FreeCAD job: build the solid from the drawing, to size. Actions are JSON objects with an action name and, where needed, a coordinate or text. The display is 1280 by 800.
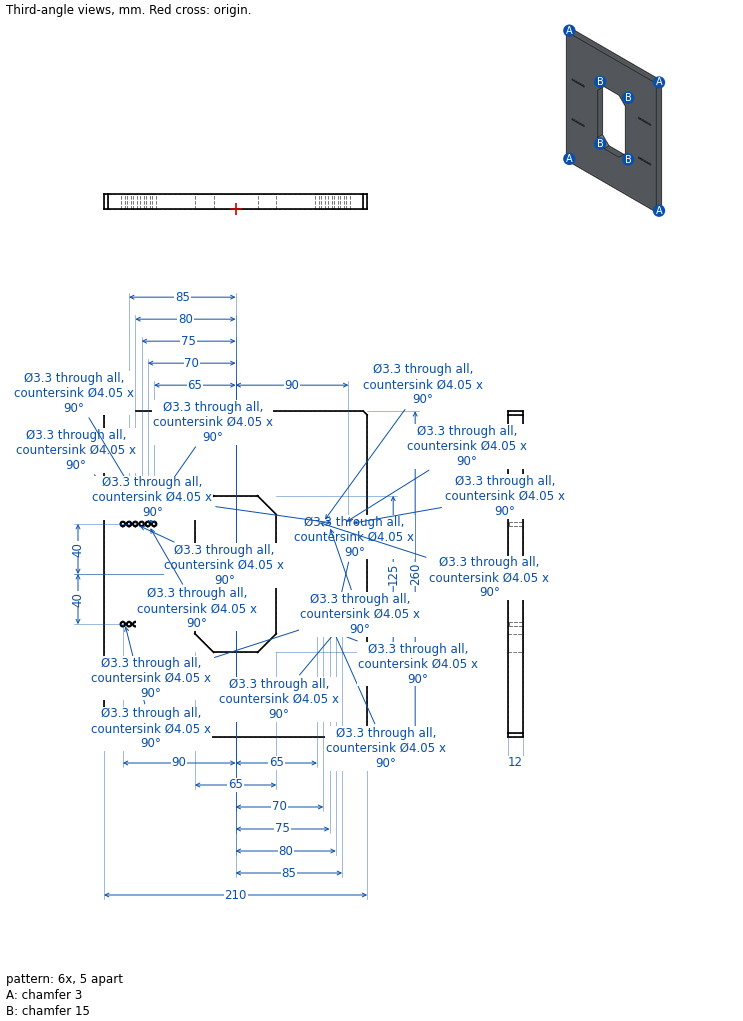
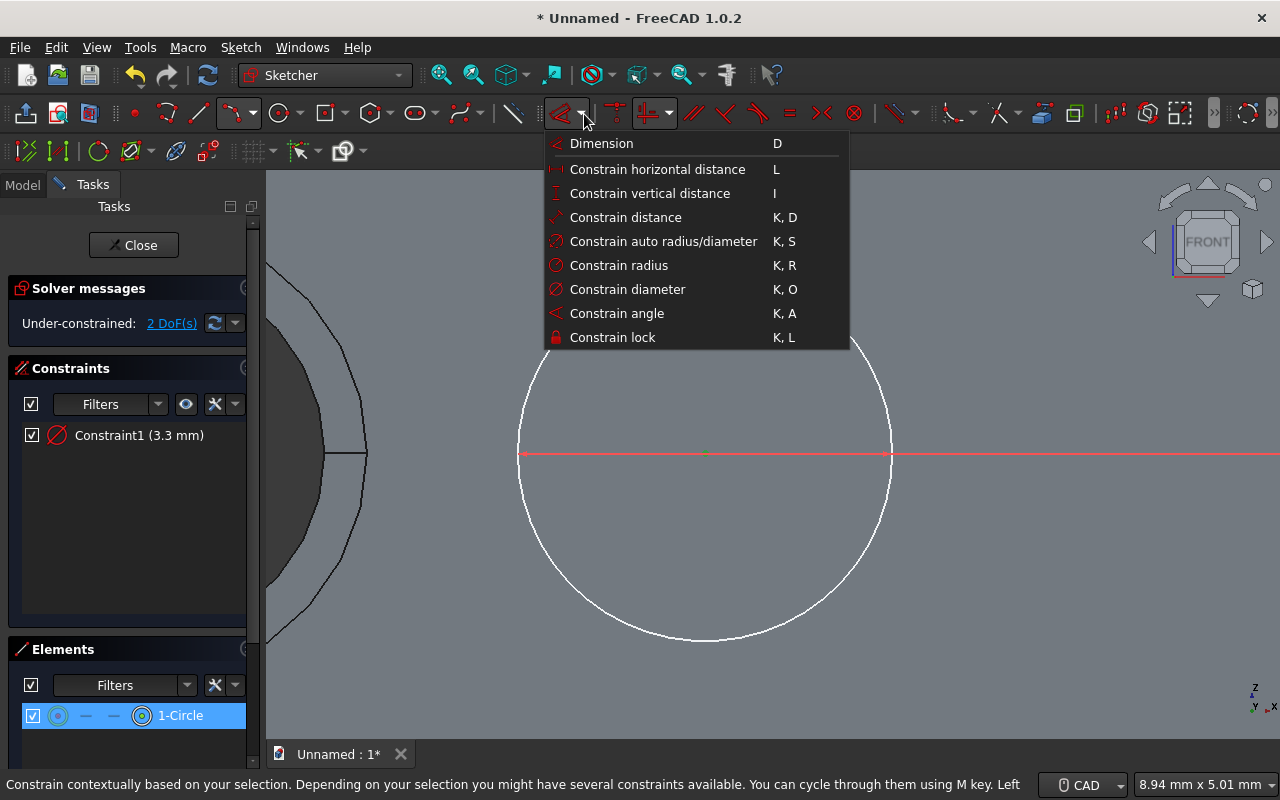
{"action": "left_click", "coordinate": [697, 169]}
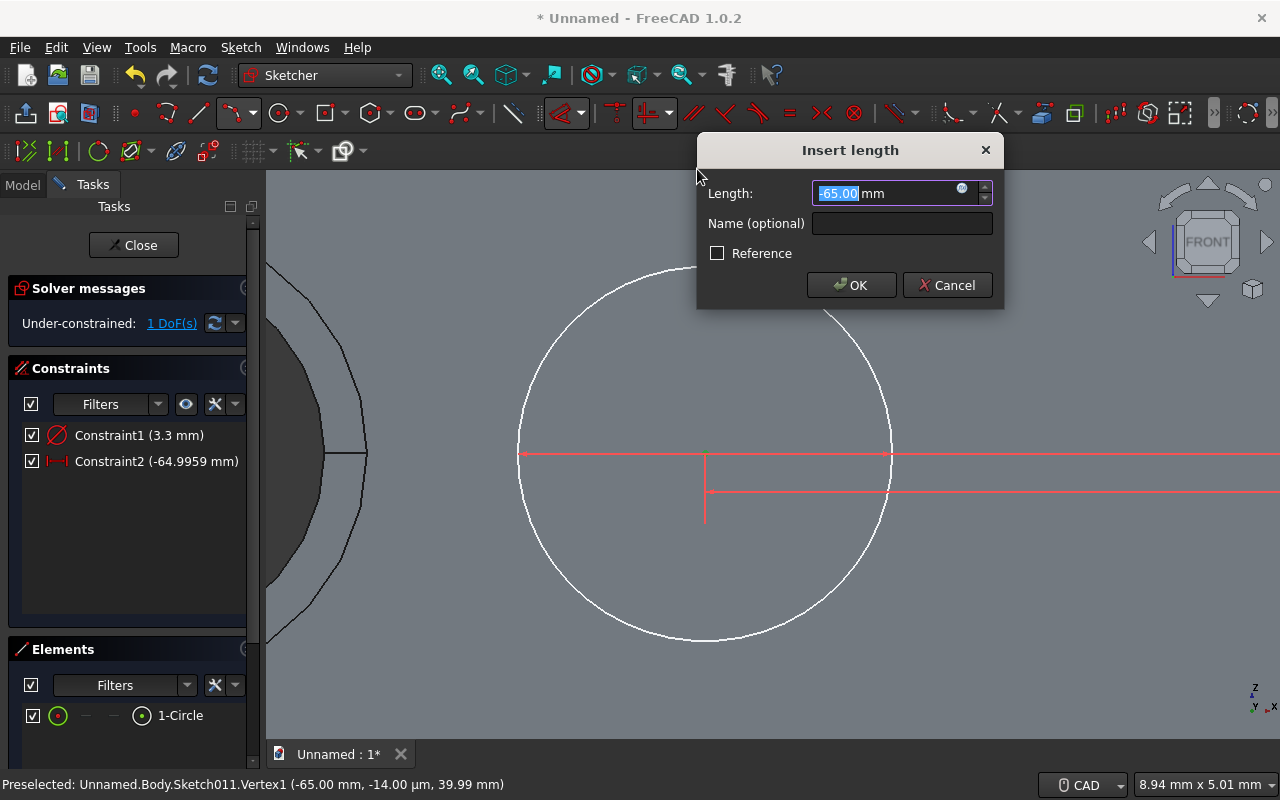
{"action": "type", "text": "-65"}
{"action": "key", "text": "Return"}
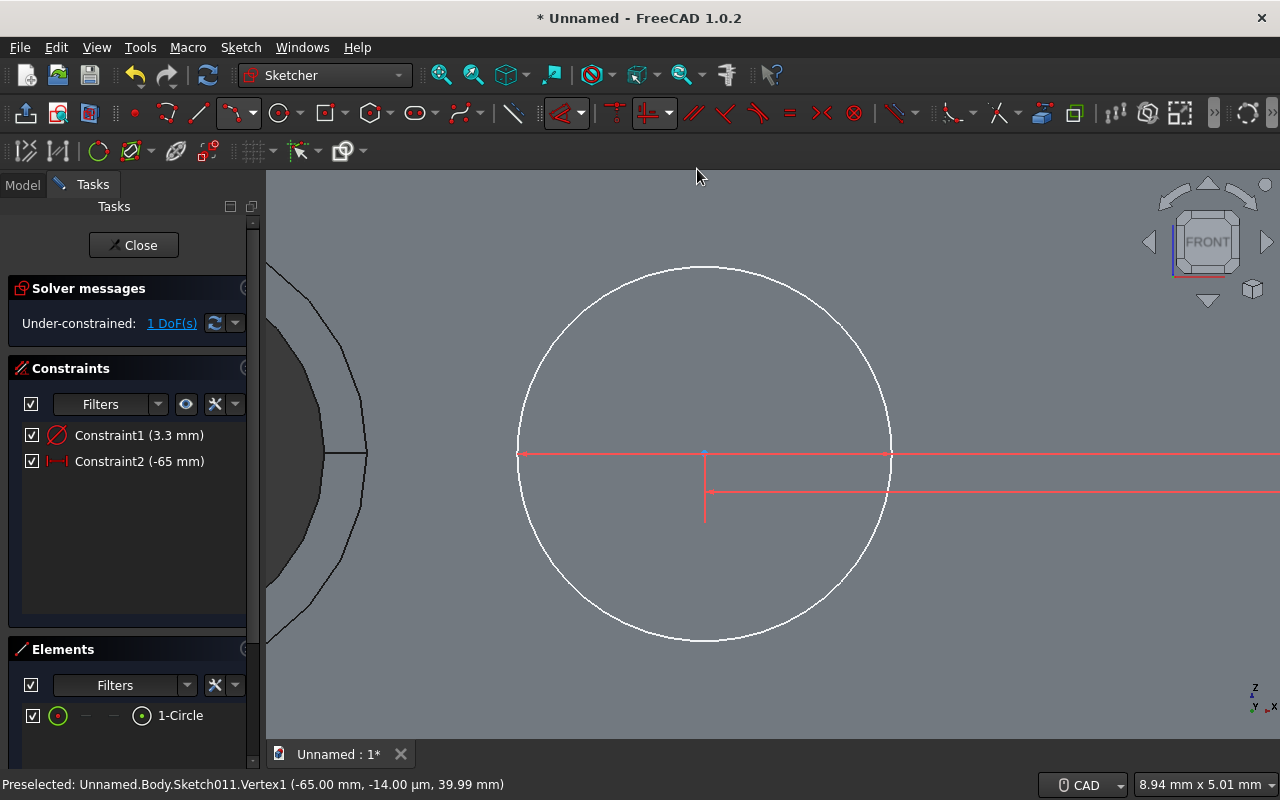
{"action": "left_click", "coordinate": [705, 454]}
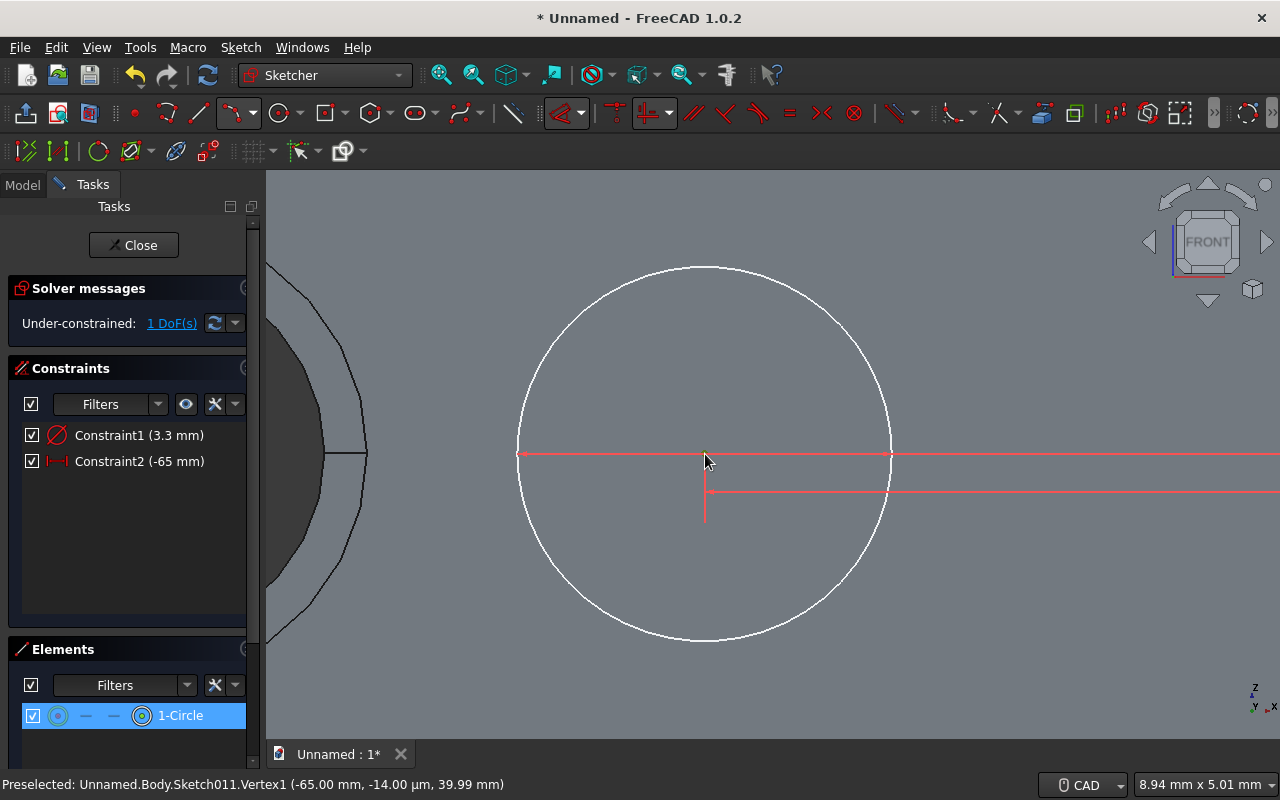
{"action": "left_click", "coordinate": [584, 114]}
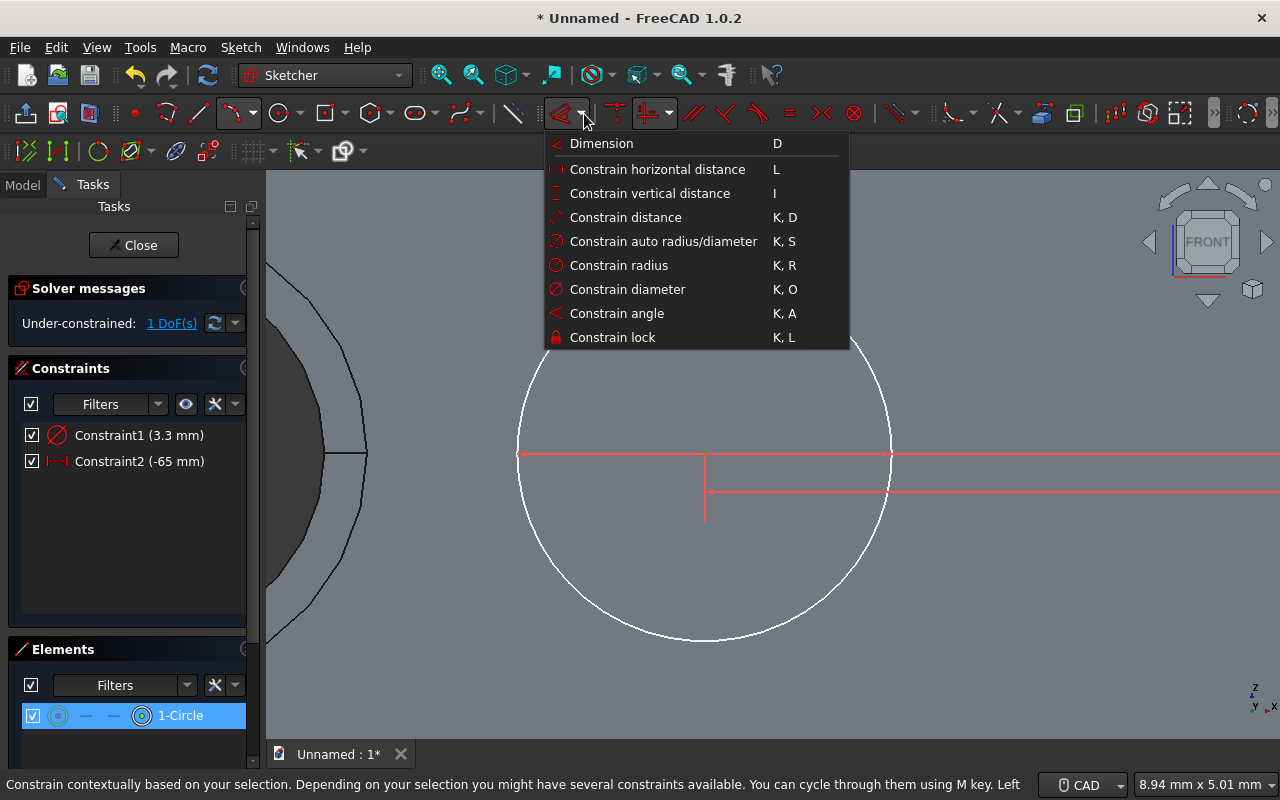
{"action": "left_click", "coordinate": [697, 193]}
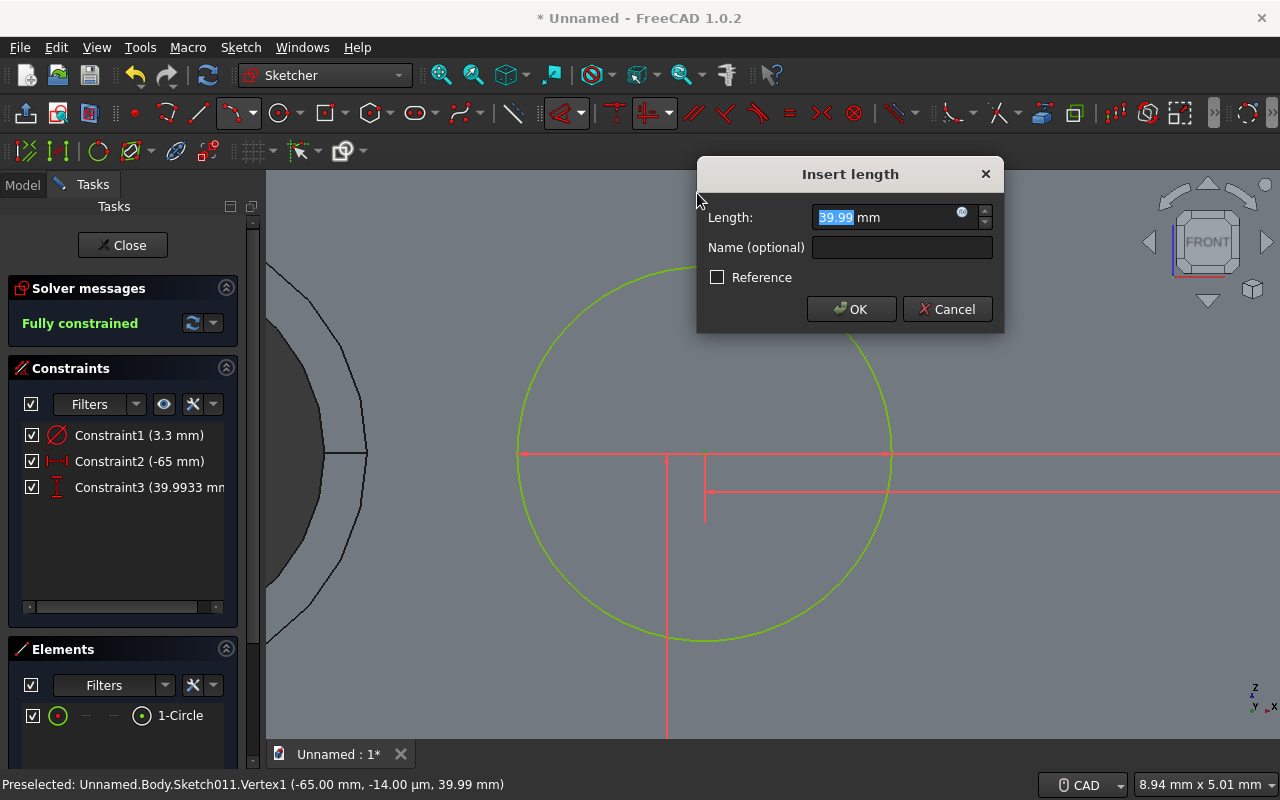
{"action": "type", "text": "40"}
{"action": "key", "text": "Return"}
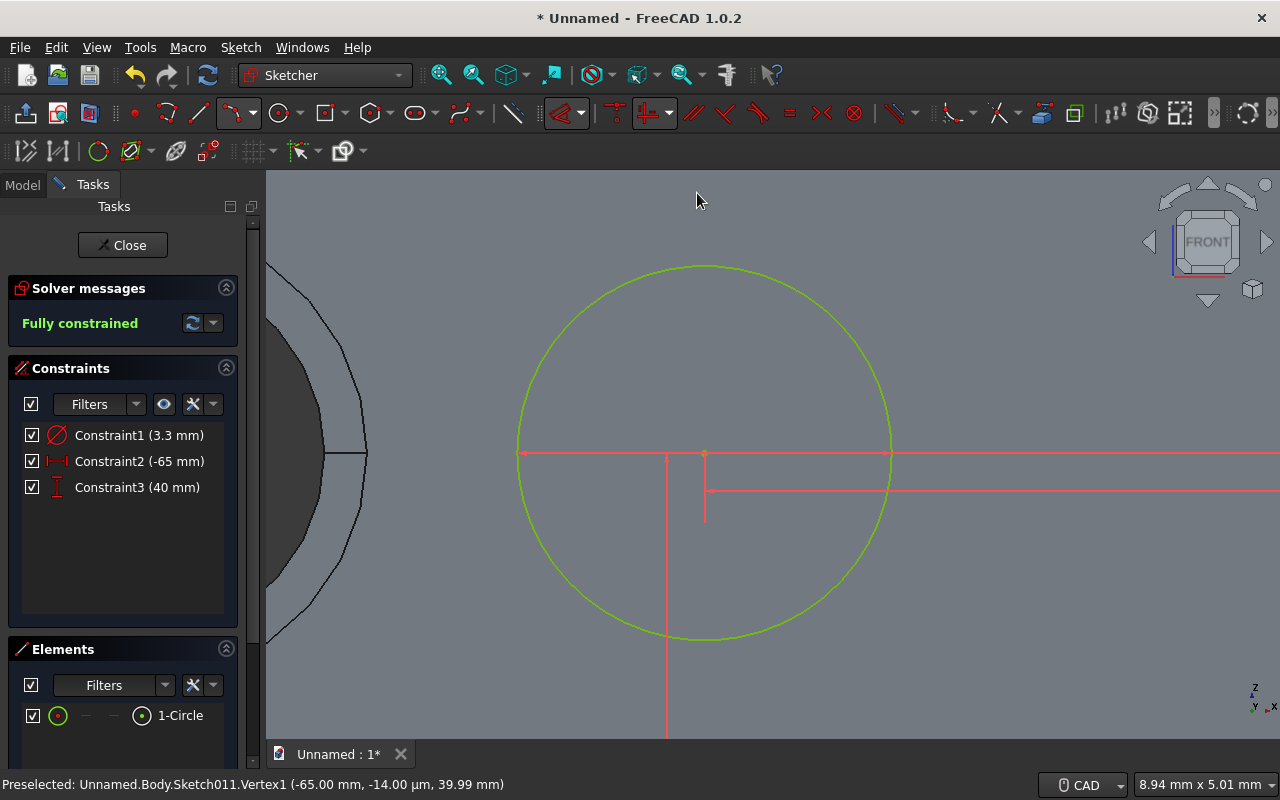
{"action": "left_click", "coordinate": [123, 245]}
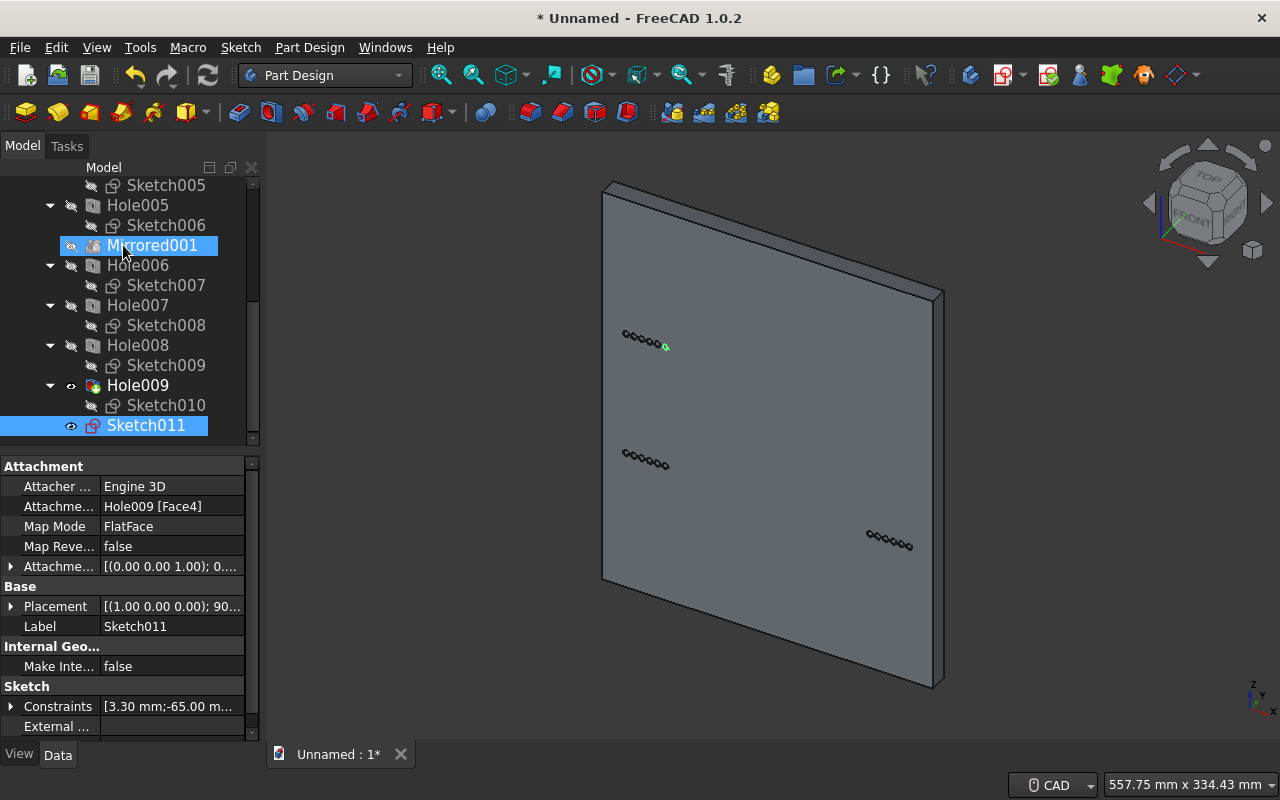
{"action": "left_click", "coordinate": [272, 112]}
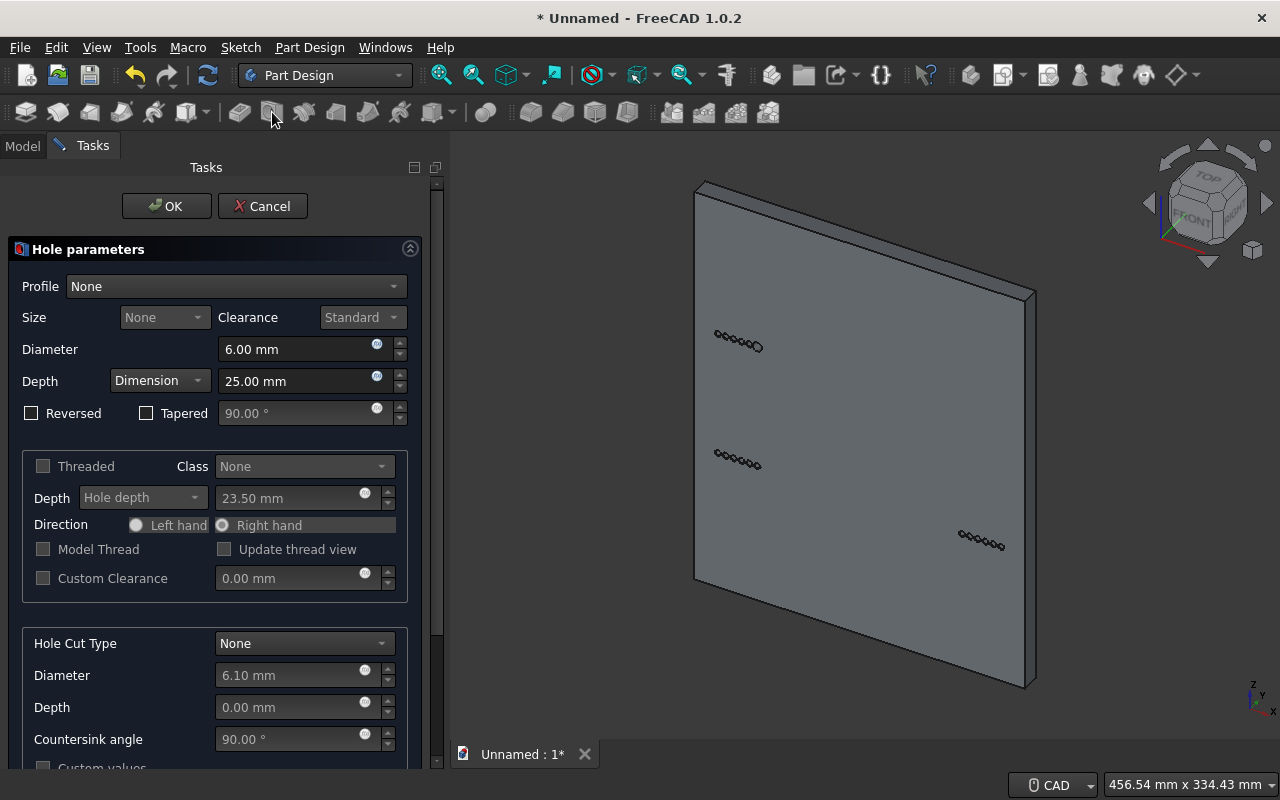
{"action": "triple_click", "coordinate": [305, 349]}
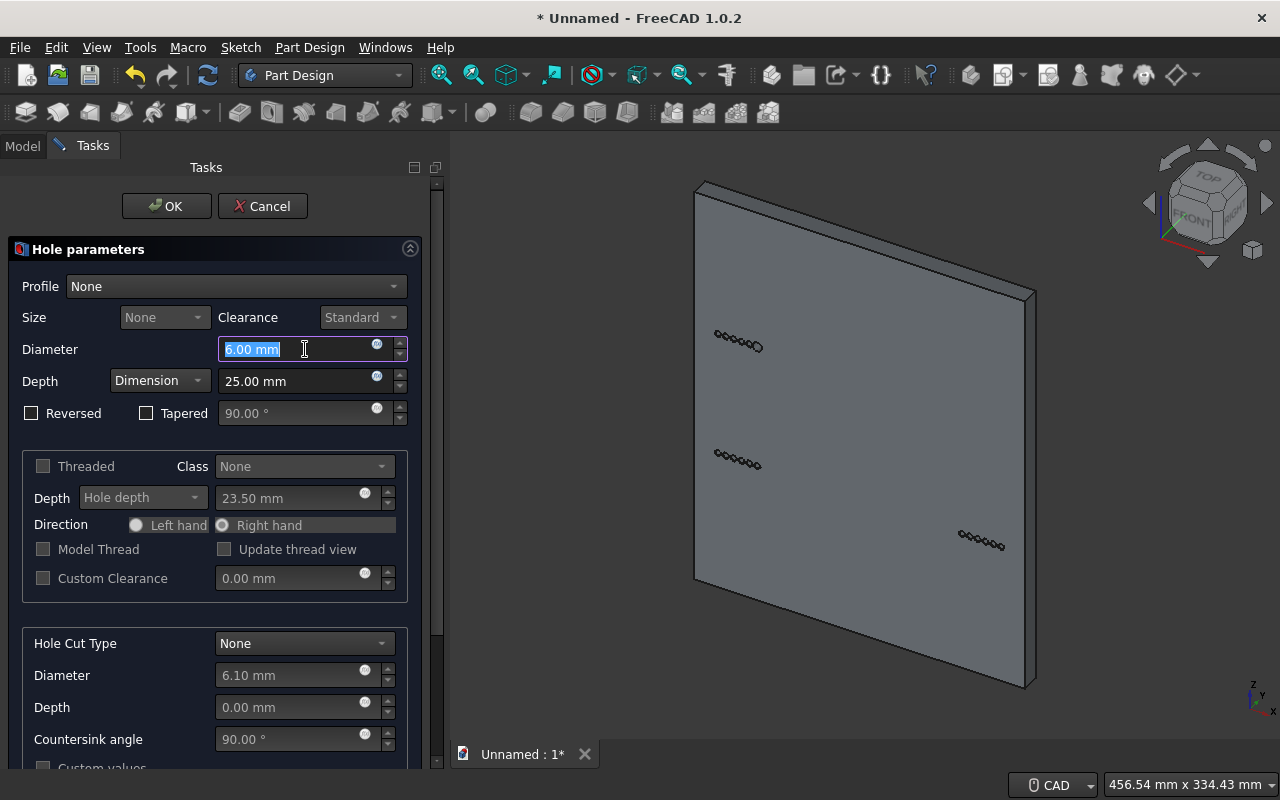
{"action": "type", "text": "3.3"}
{"action": "key", "text": "Tab"}